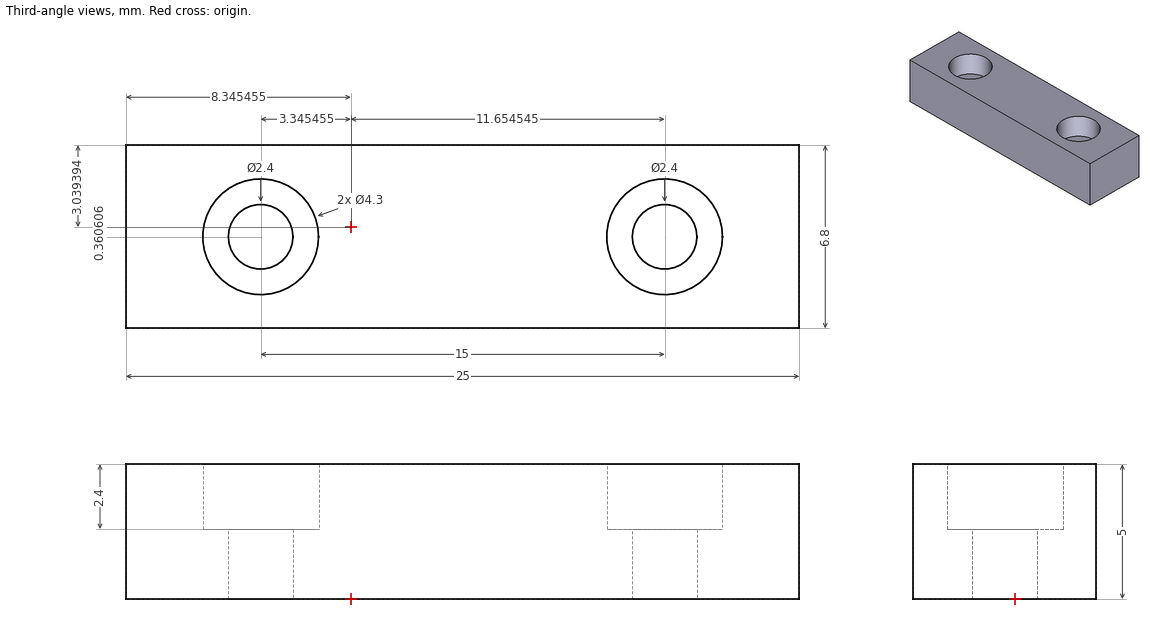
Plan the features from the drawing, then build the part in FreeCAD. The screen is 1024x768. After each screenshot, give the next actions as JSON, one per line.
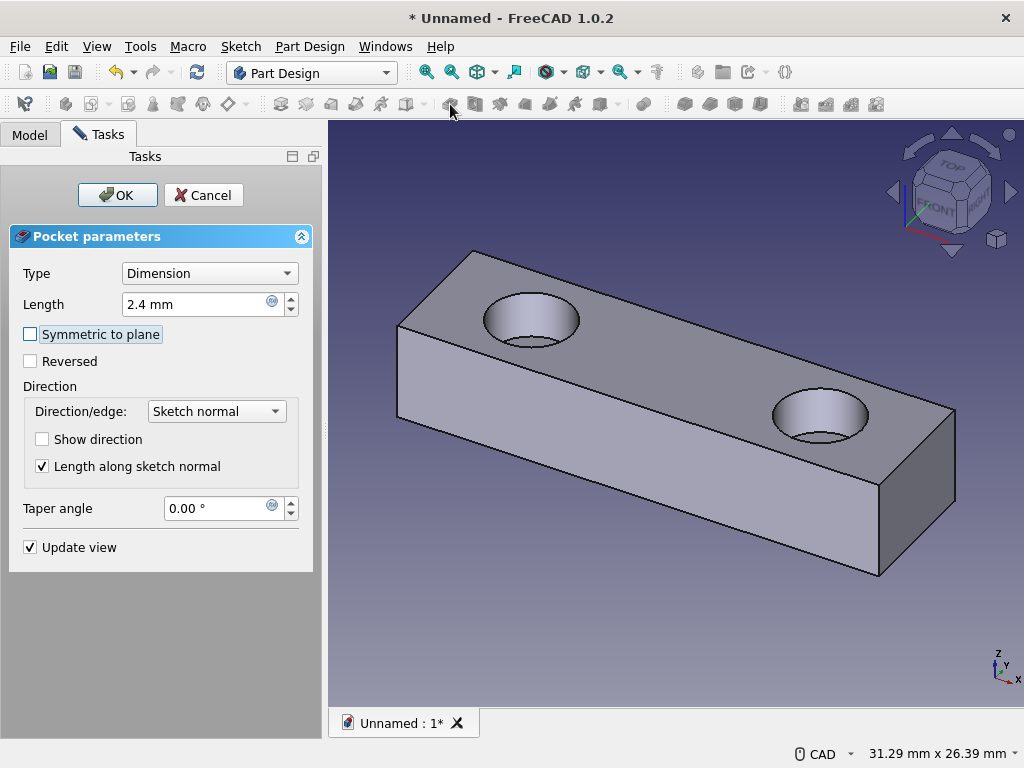
{"action": "left_click", "coordinate": [118, 195]}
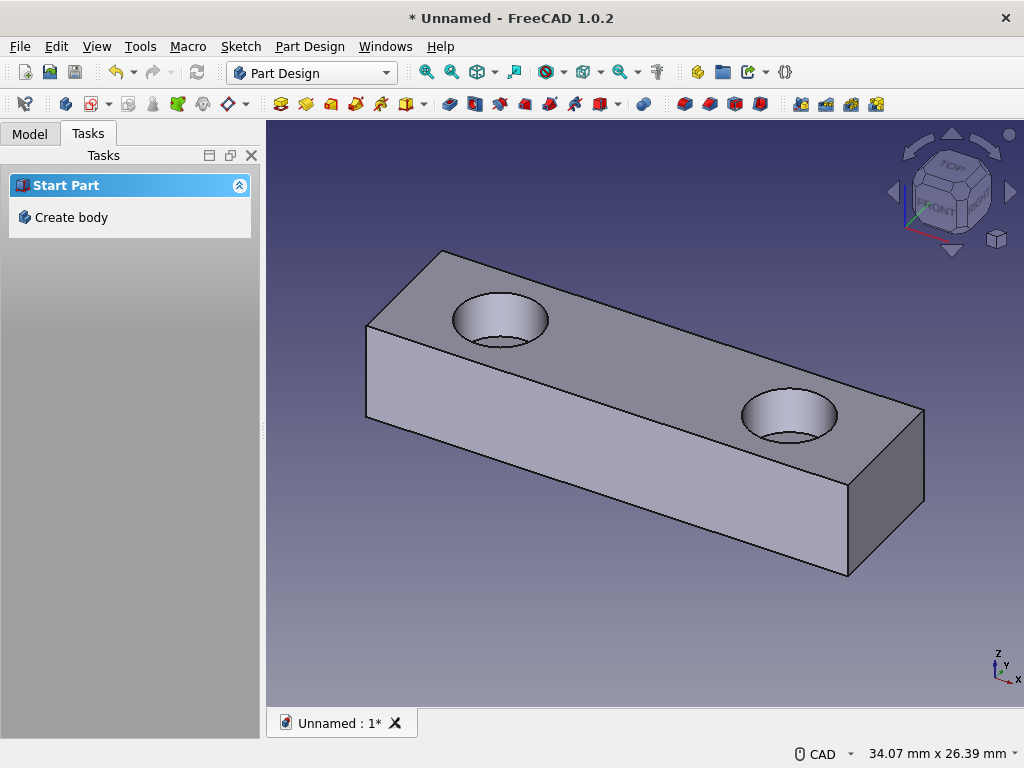
{"action": "key", "text": "0"}